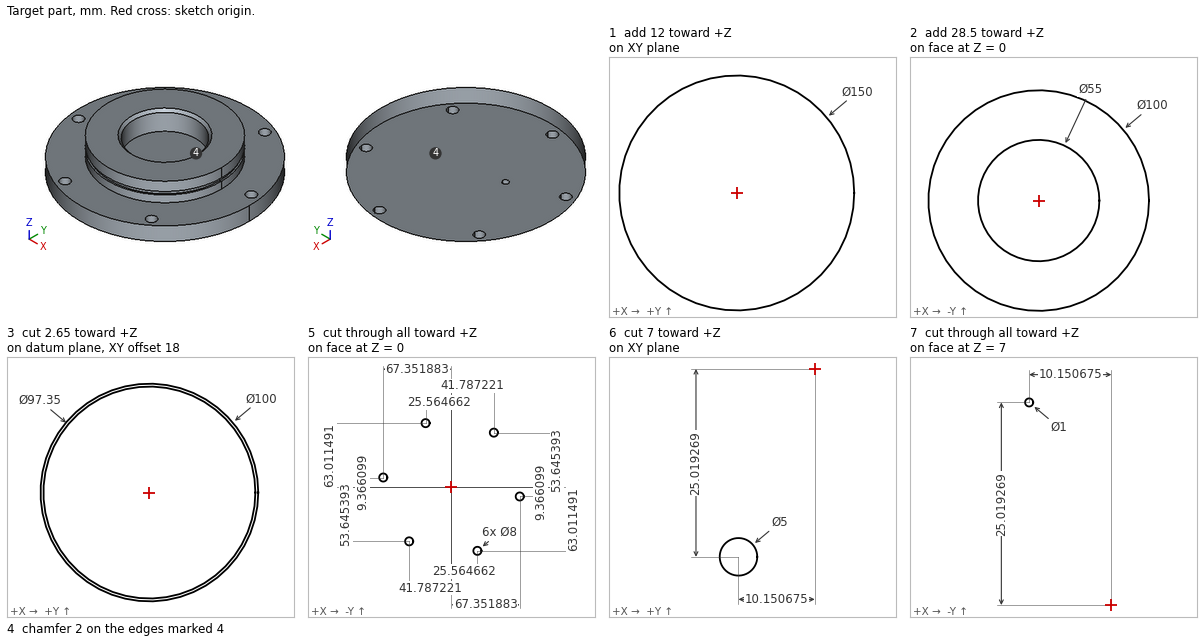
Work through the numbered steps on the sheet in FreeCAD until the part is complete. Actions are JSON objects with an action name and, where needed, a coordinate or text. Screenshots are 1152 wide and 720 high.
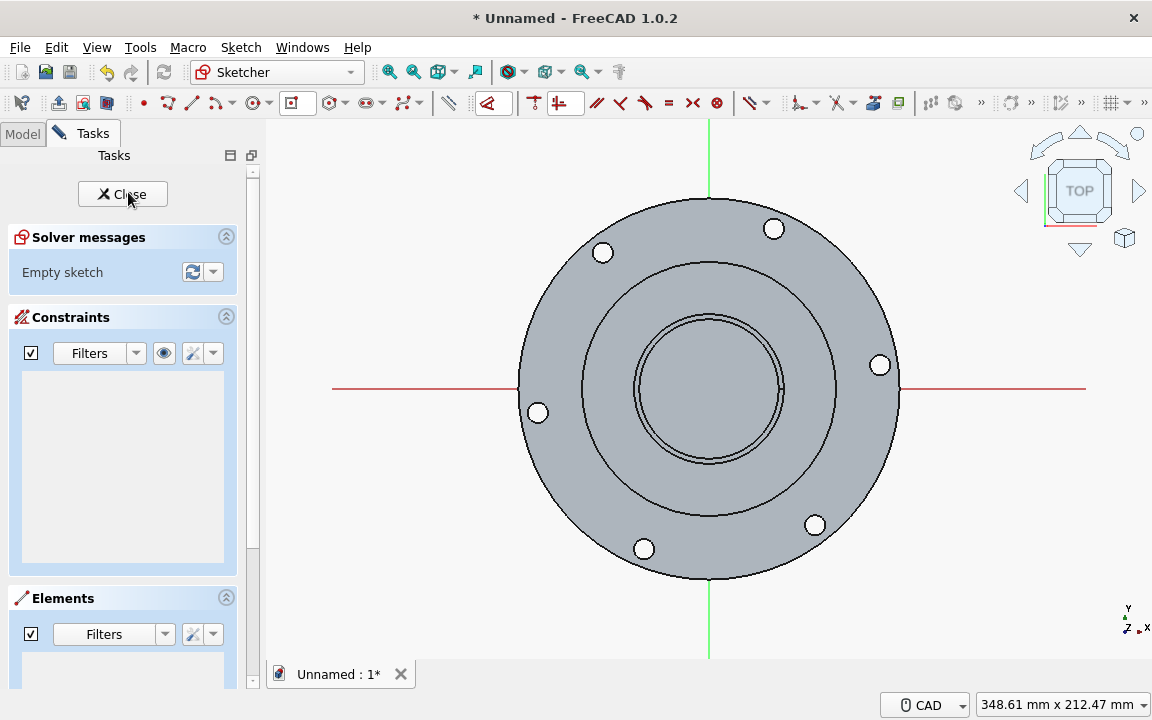
{"action": "left_click", "coordinate": [108, 104]}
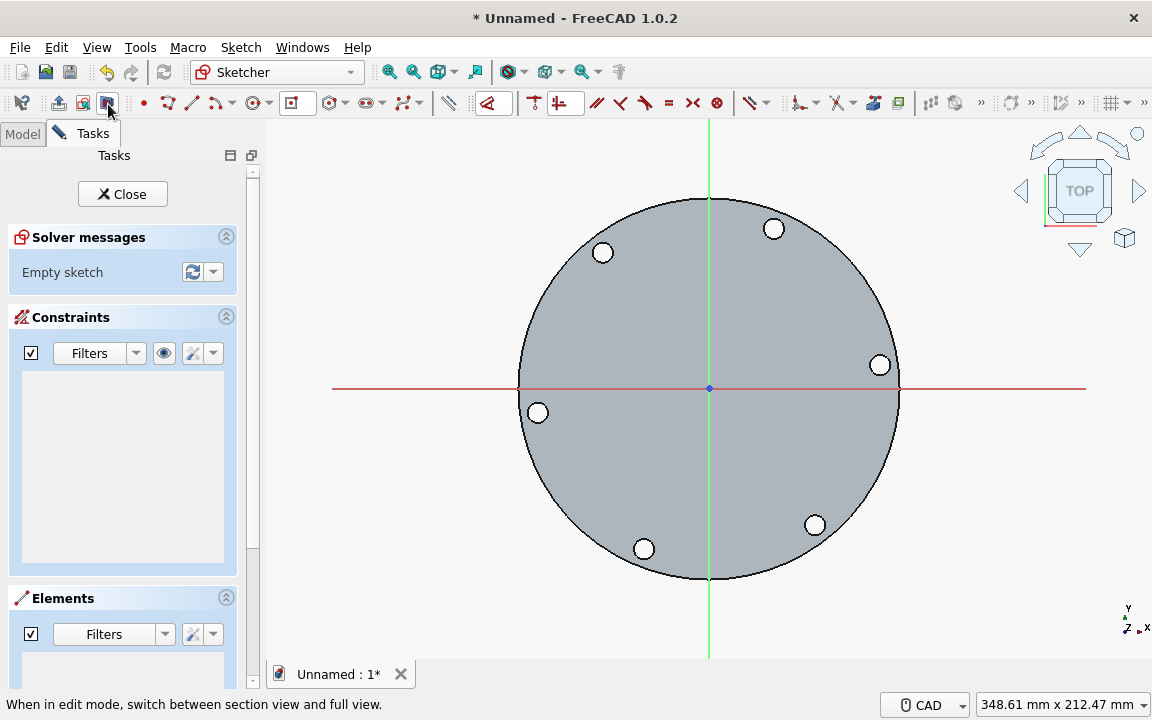
{"action": "scroll", "coordinate": [685, 456], "scroll_direction": "up", "scroll_amount": 15}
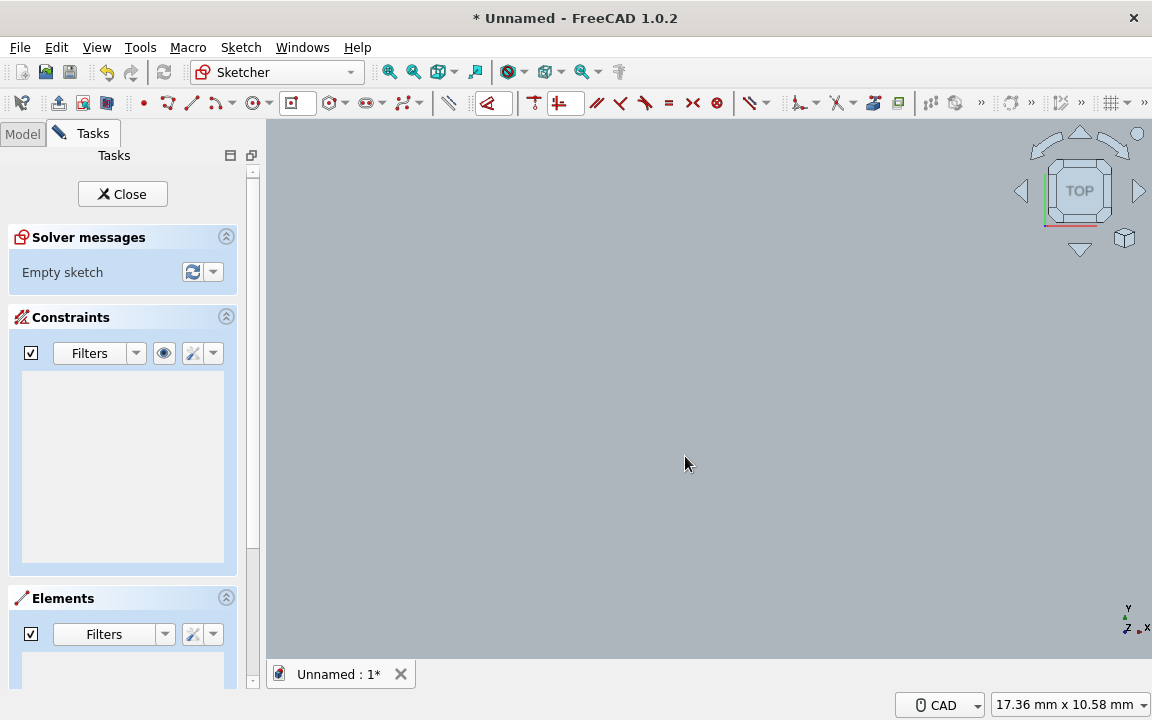
{"action": "left_click", "coordinate": [254, 104]}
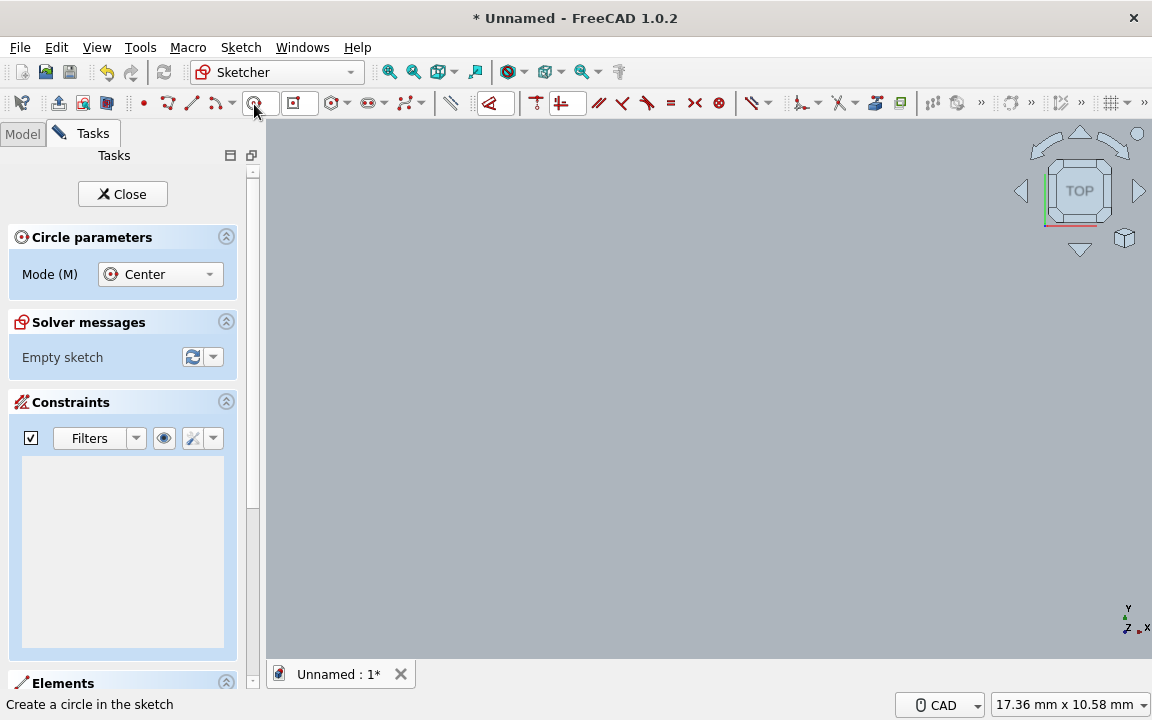
{"action": "left_click", "coordinate": [640, 376]}
{"action": "mouse_move", "coordinate": [730, 285]}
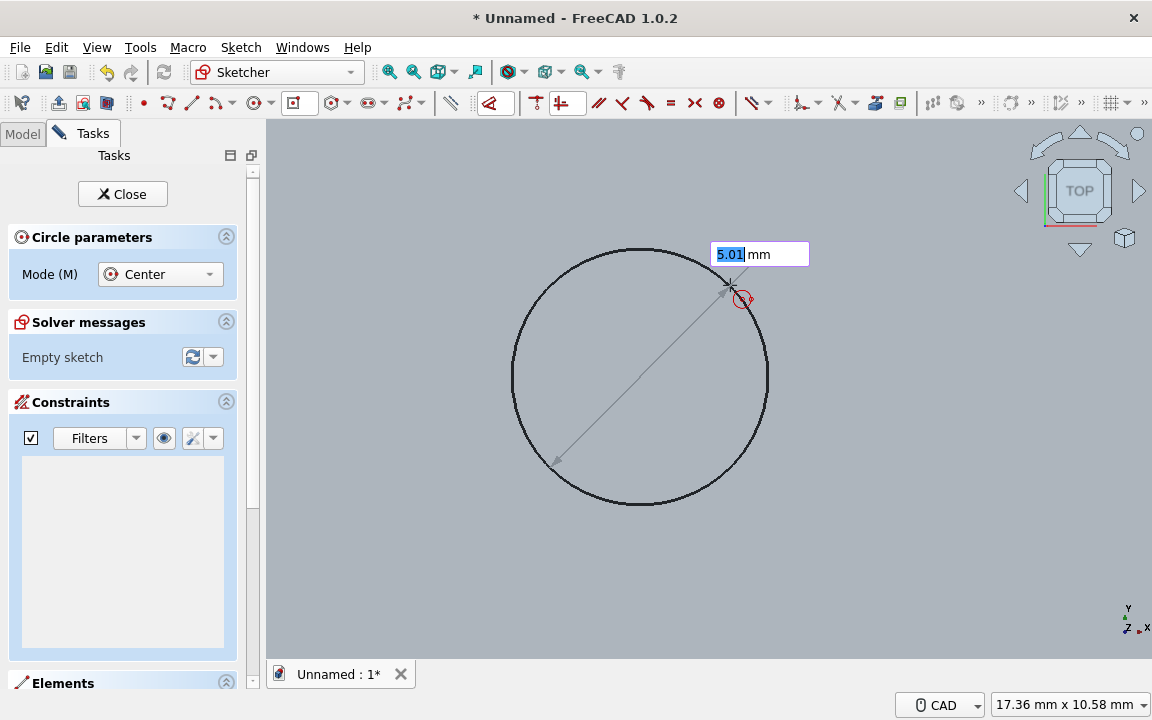
{"action": "type", "text": "5"}
{"action": "key", "text": "Return"}
{"action": "key", "text": "Escape"}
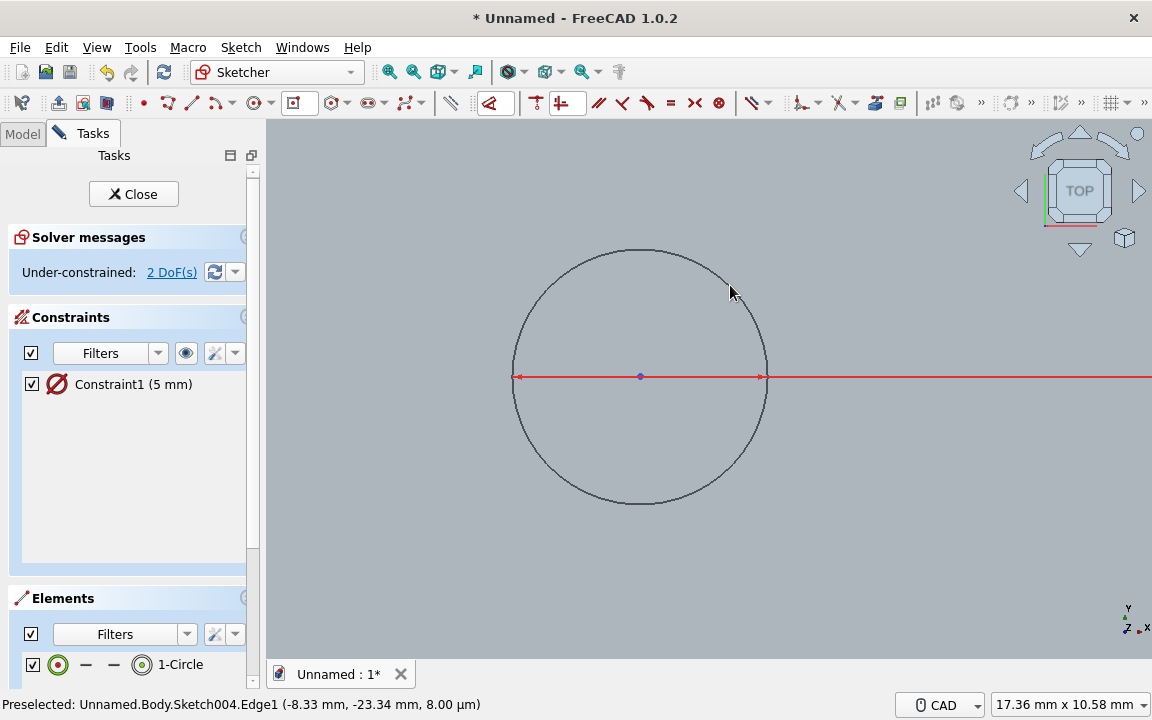
{"action": "left_click", "coordinate": [640, 377]}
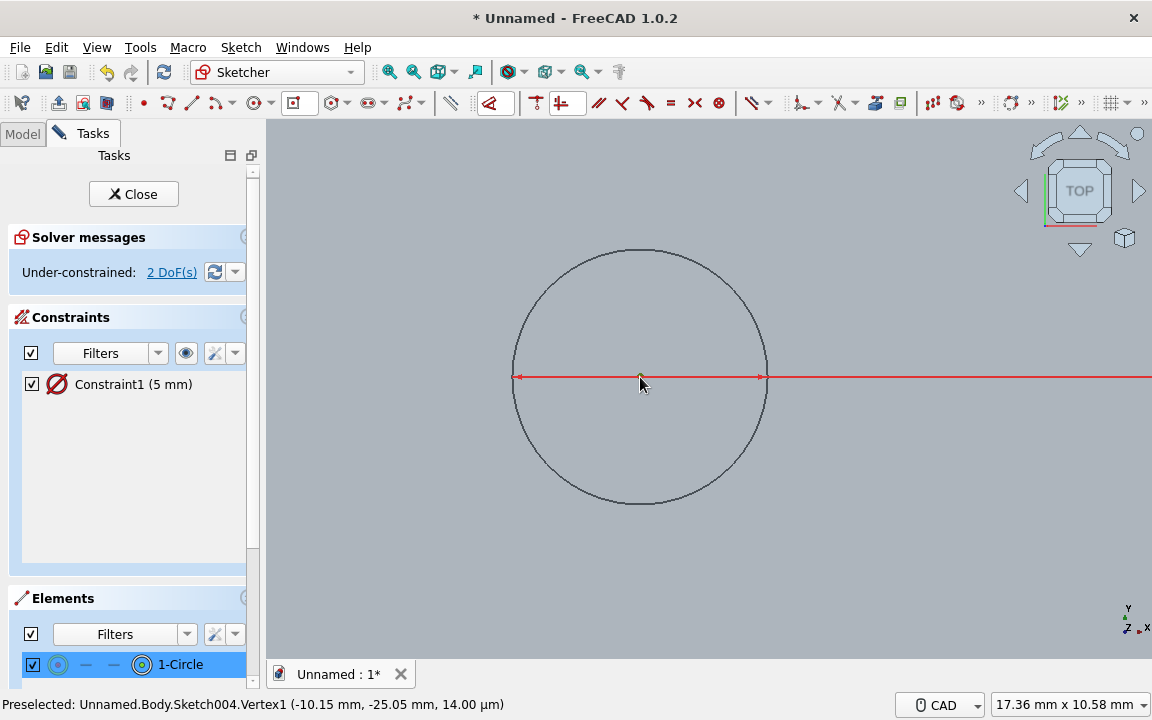
{"action": "key", "text": "l"}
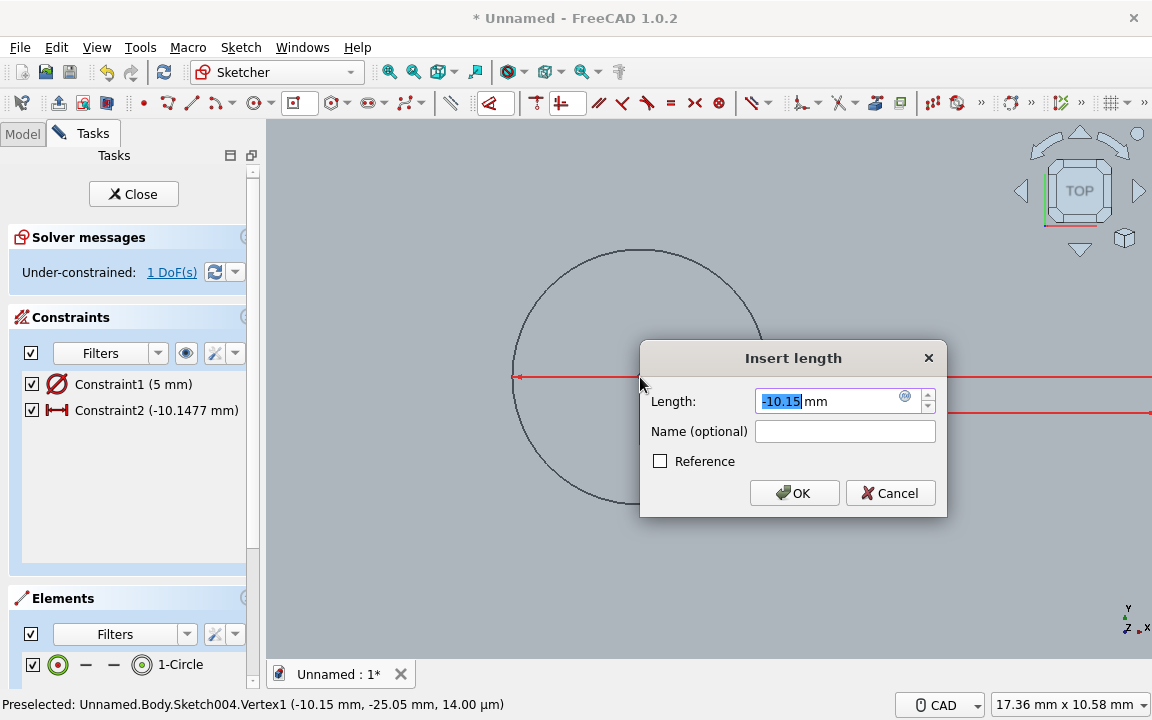
{"action": "type", "text": "-10.150675"}
{"action": "key", "text": "Return"}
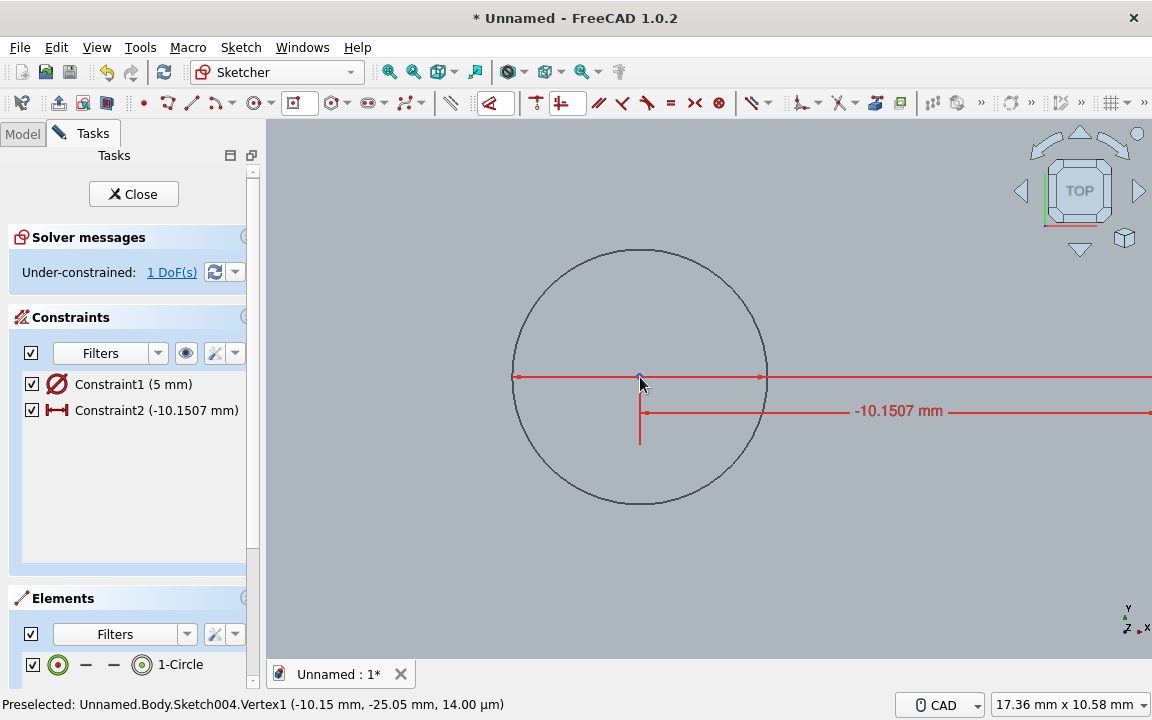
{"action": "left_click", "coordinate": [640, 377]}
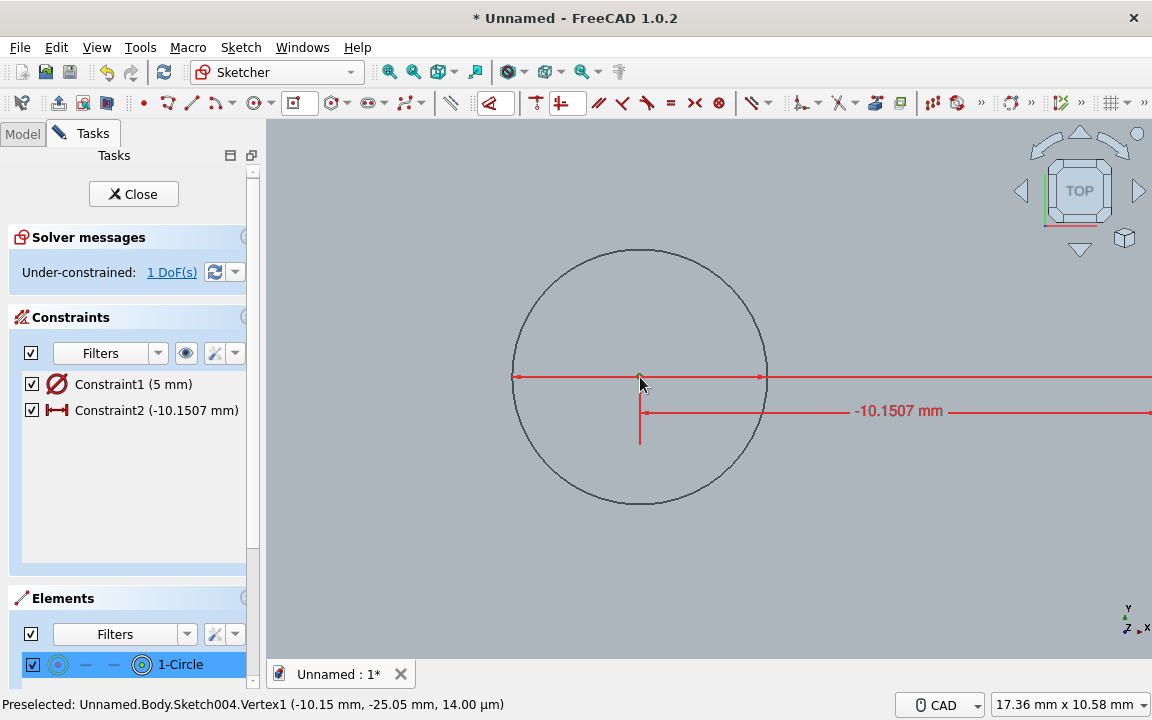
{"action": "left_click", "coordinate": [508, 104]}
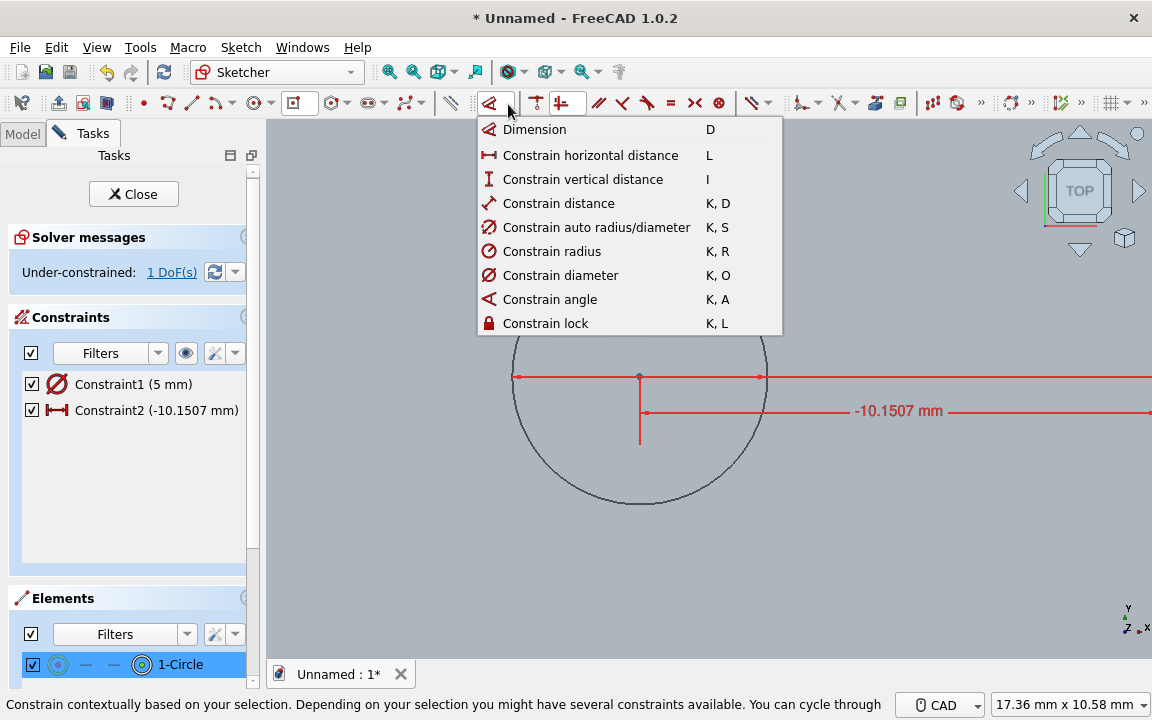
{"action": "left_click", "coordinate": [630, 179]}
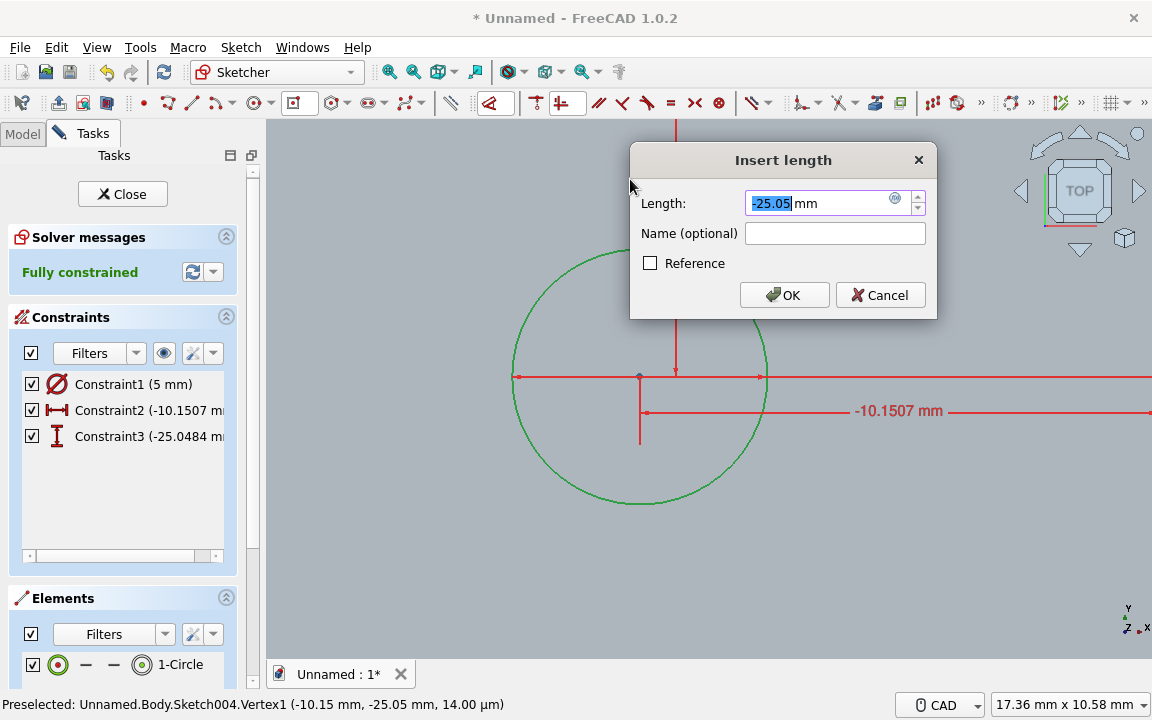
{"action": "type", "text": "-25.019269"}
{"action": "key", "text": "Return"}